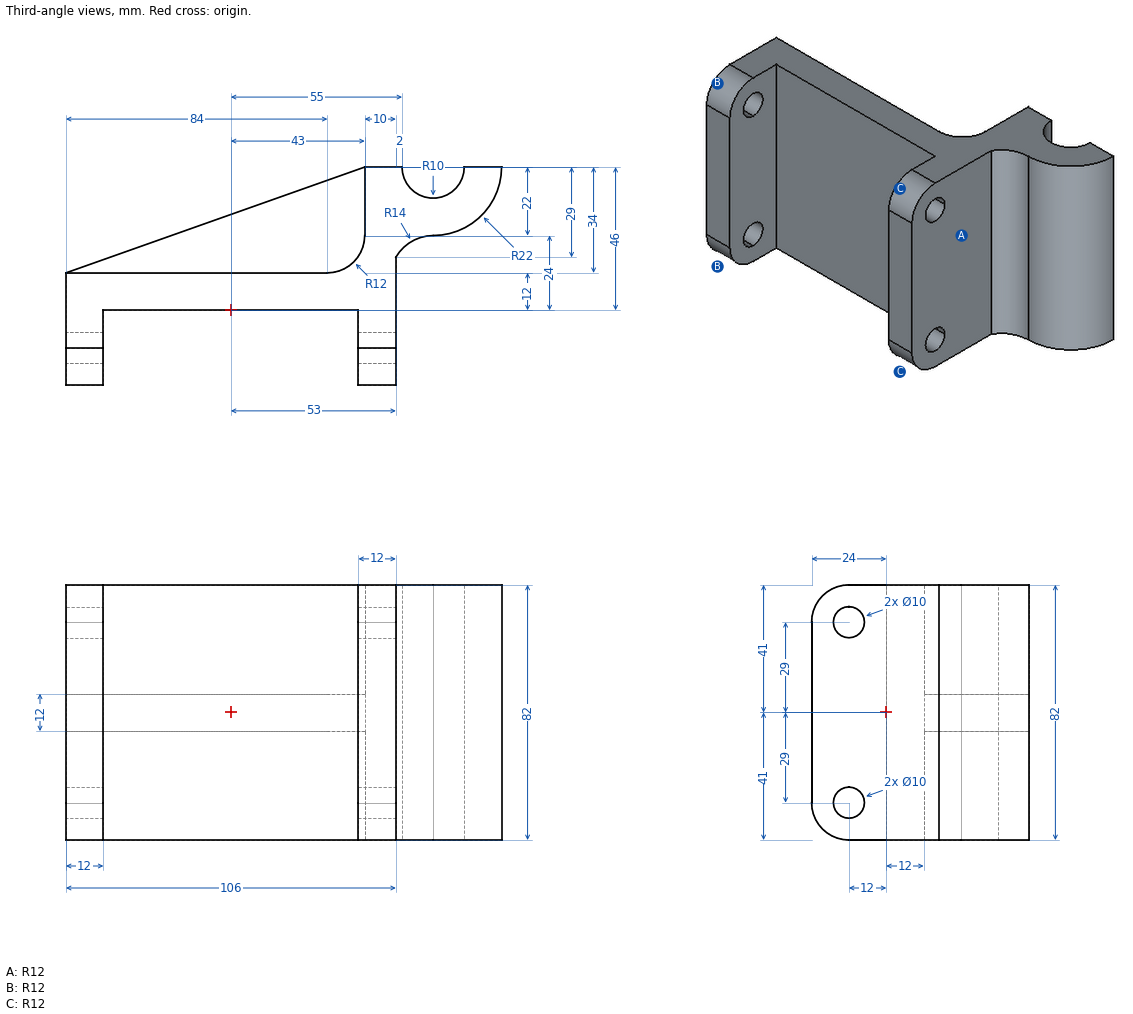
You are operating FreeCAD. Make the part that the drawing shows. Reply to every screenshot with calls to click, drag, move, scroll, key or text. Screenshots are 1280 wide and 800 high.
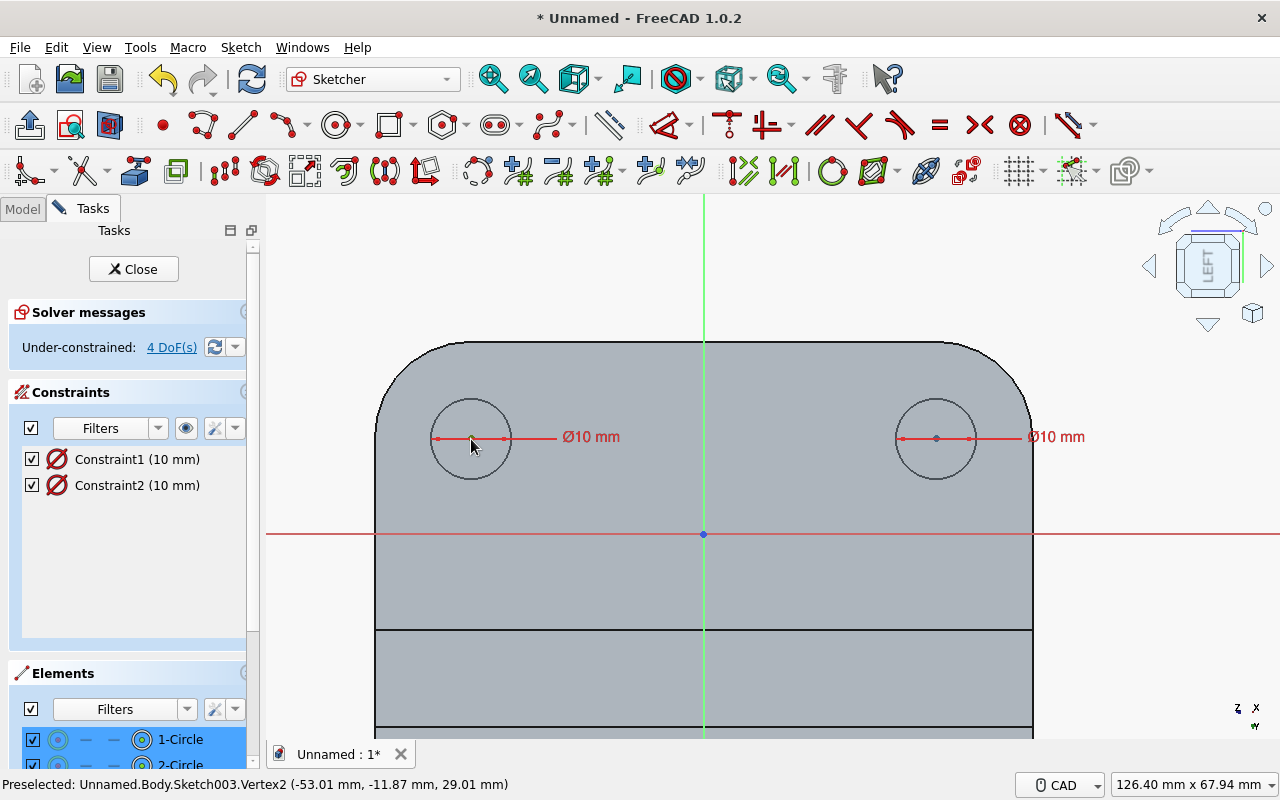
key(h)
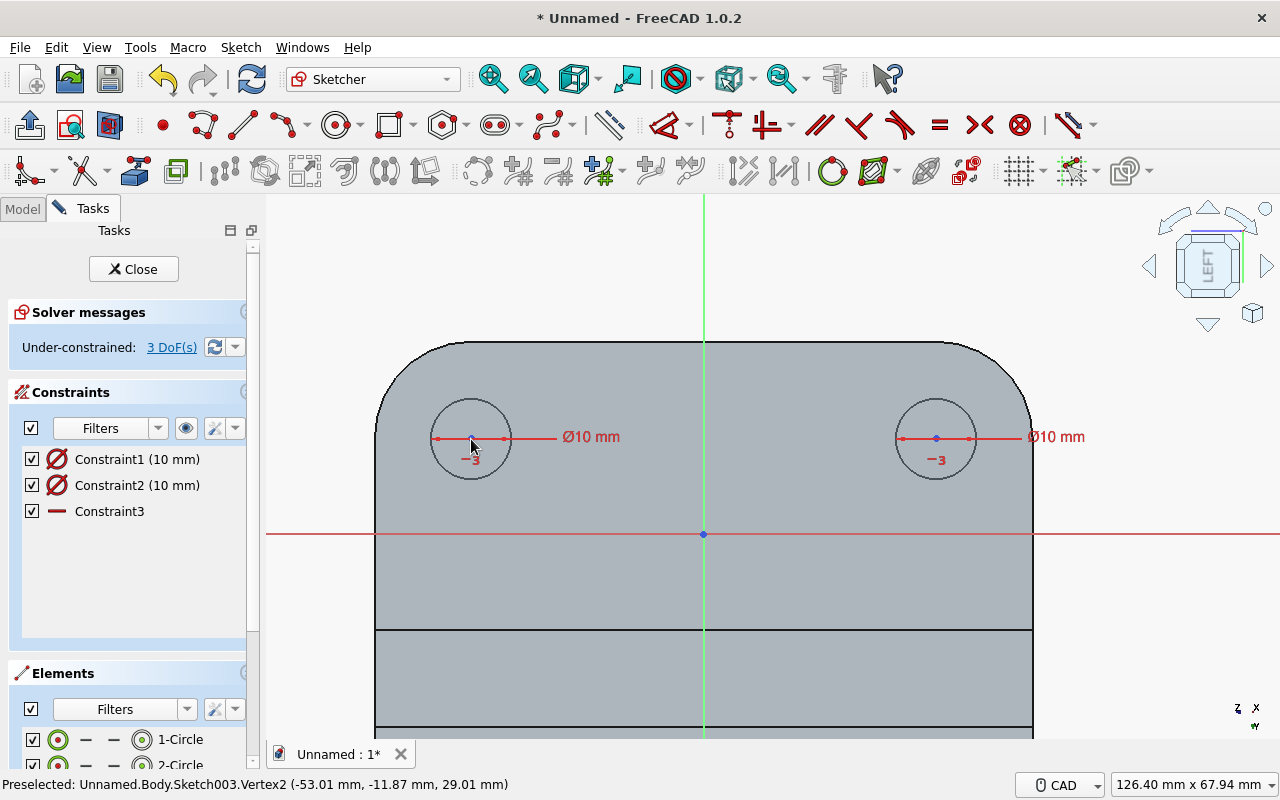
key(d)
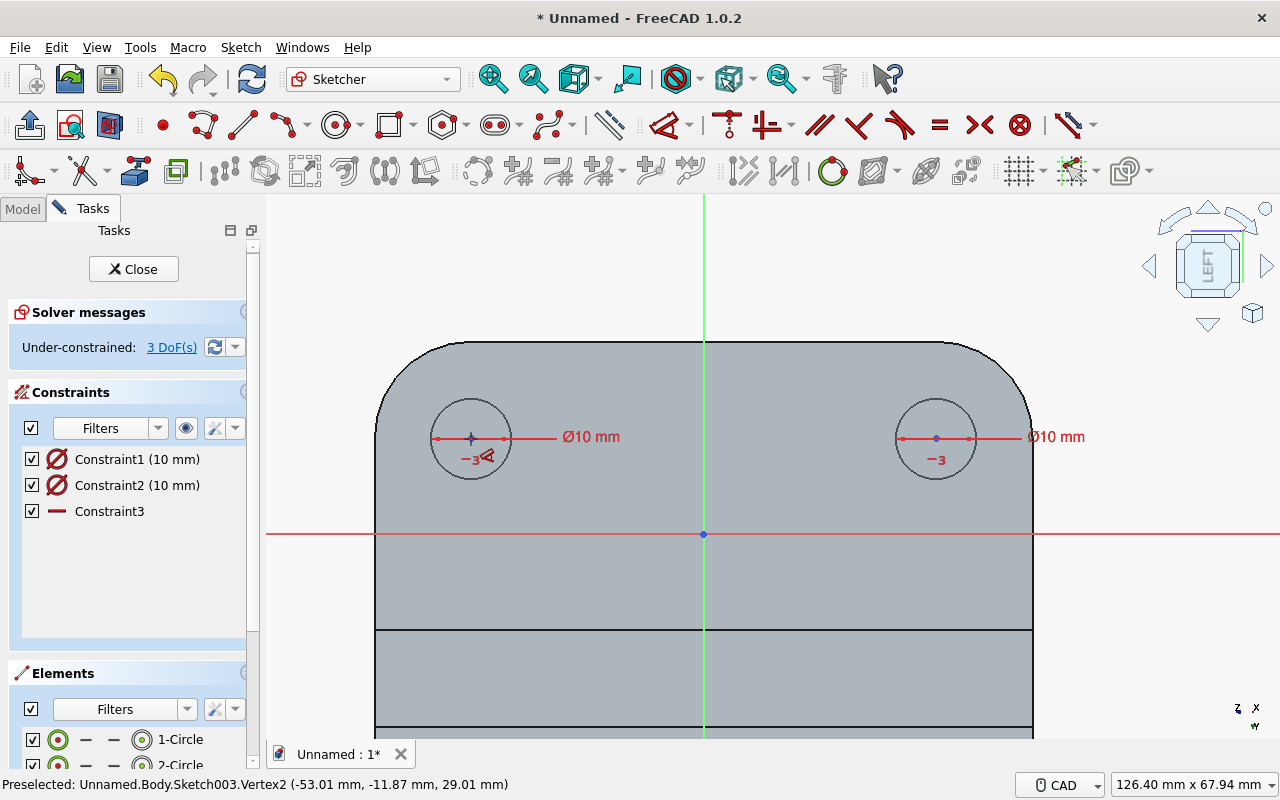
click(936, 439)
click(820, 568)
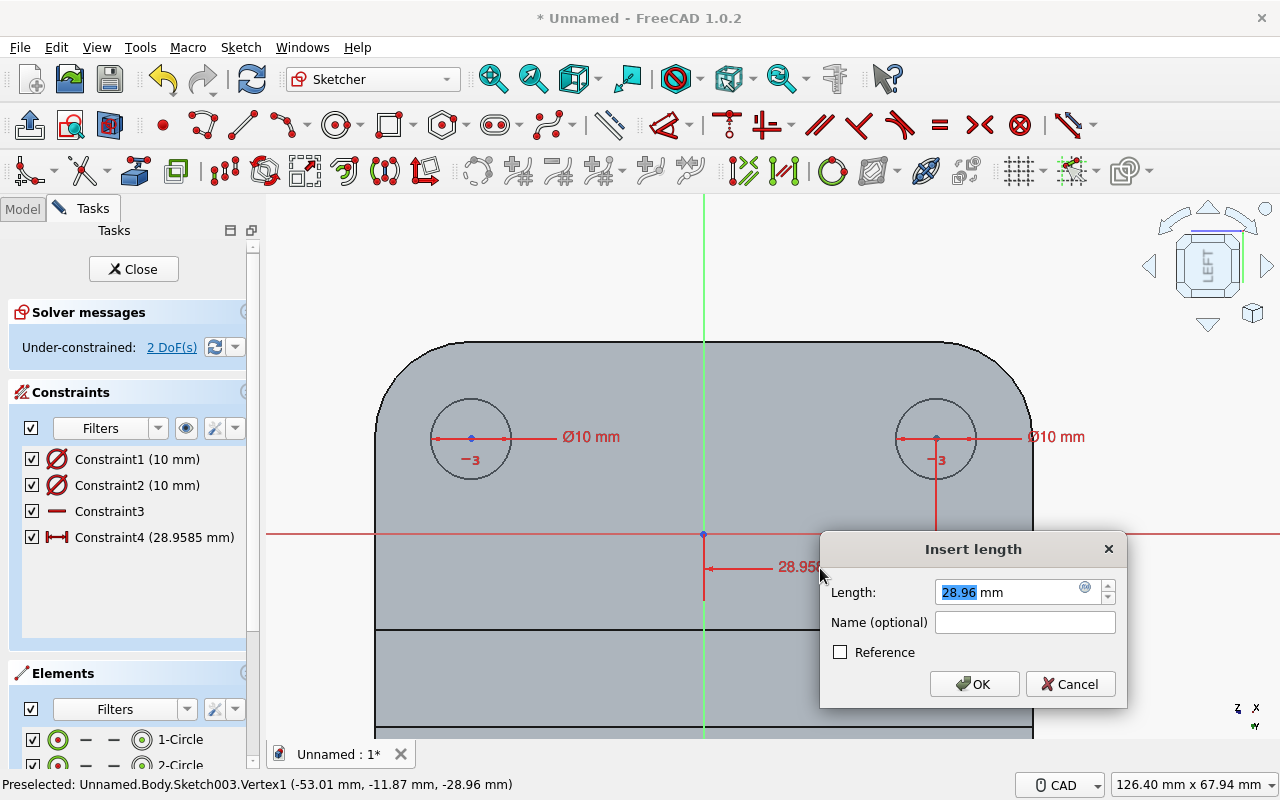
text(29)
key(Return)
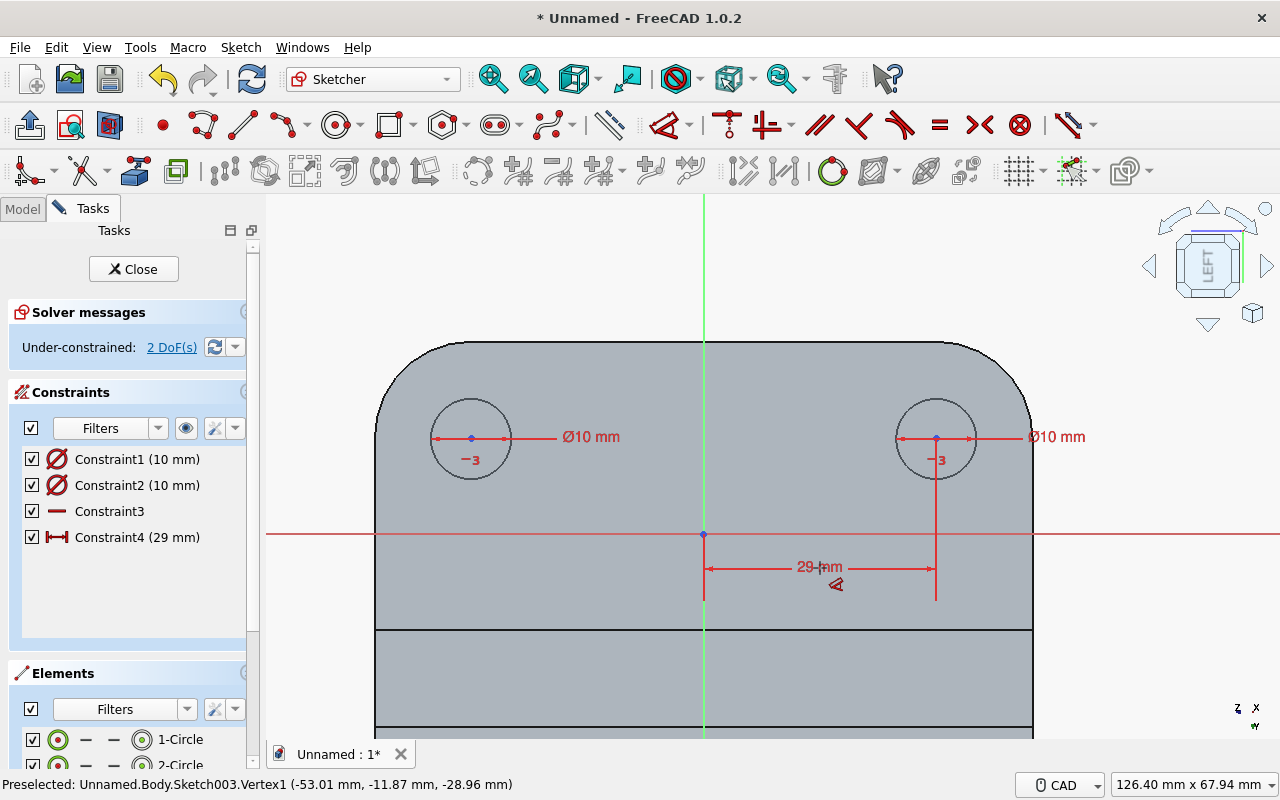
click(936, 439)
click(970, 487)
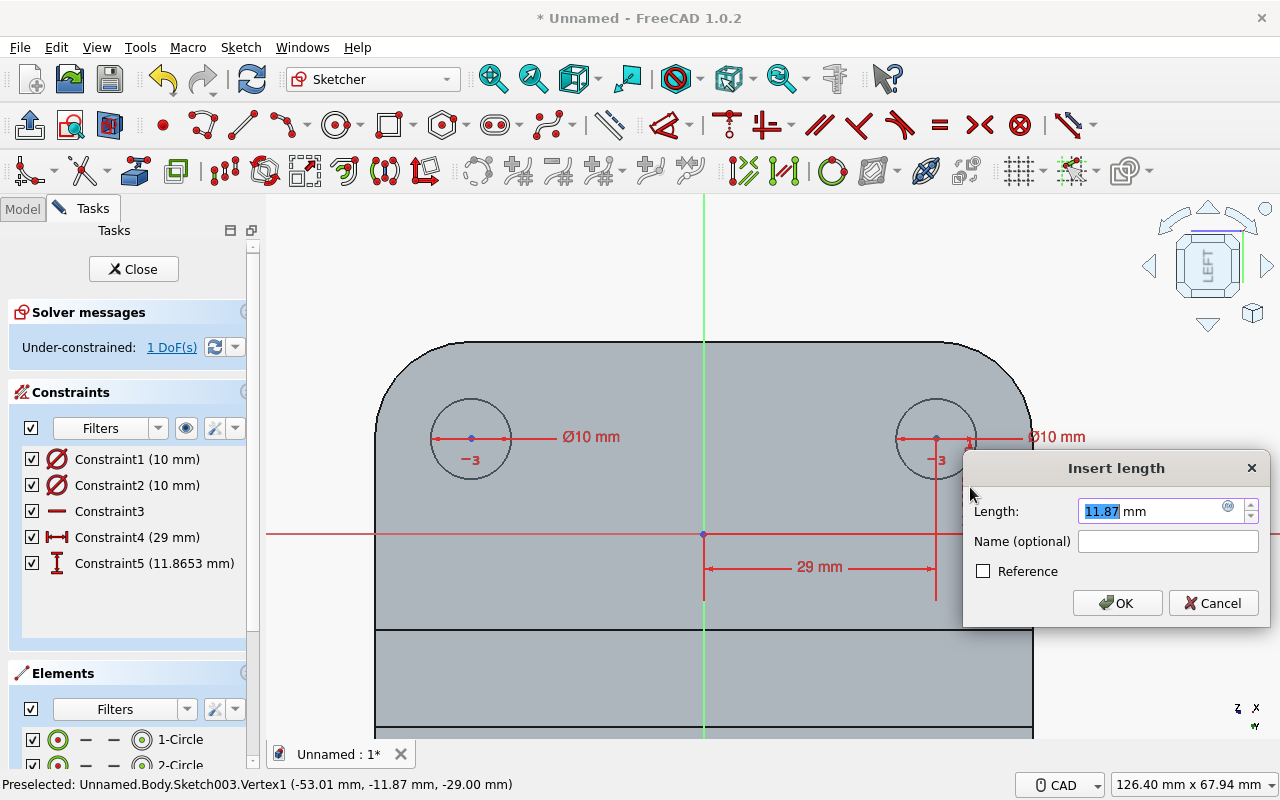
text(12)
key(Return)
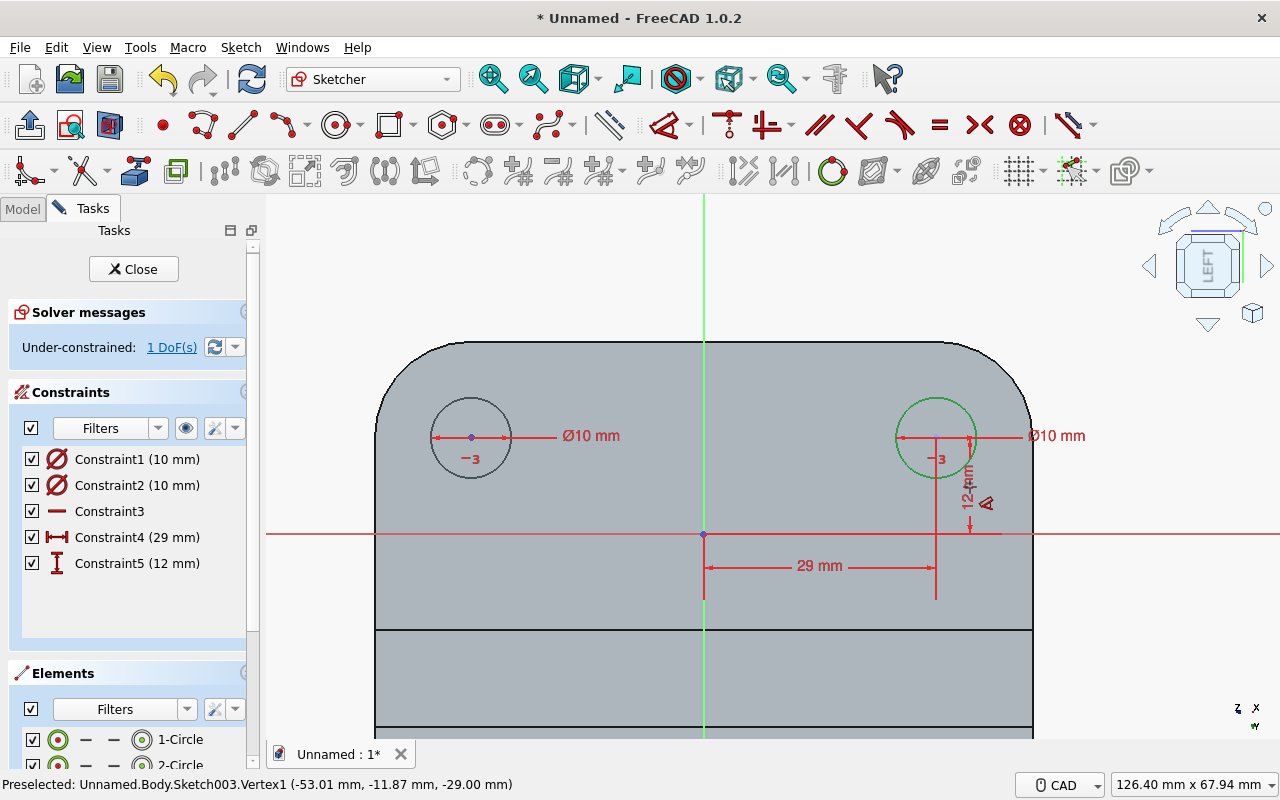
click(471, 438)
click(587, 568)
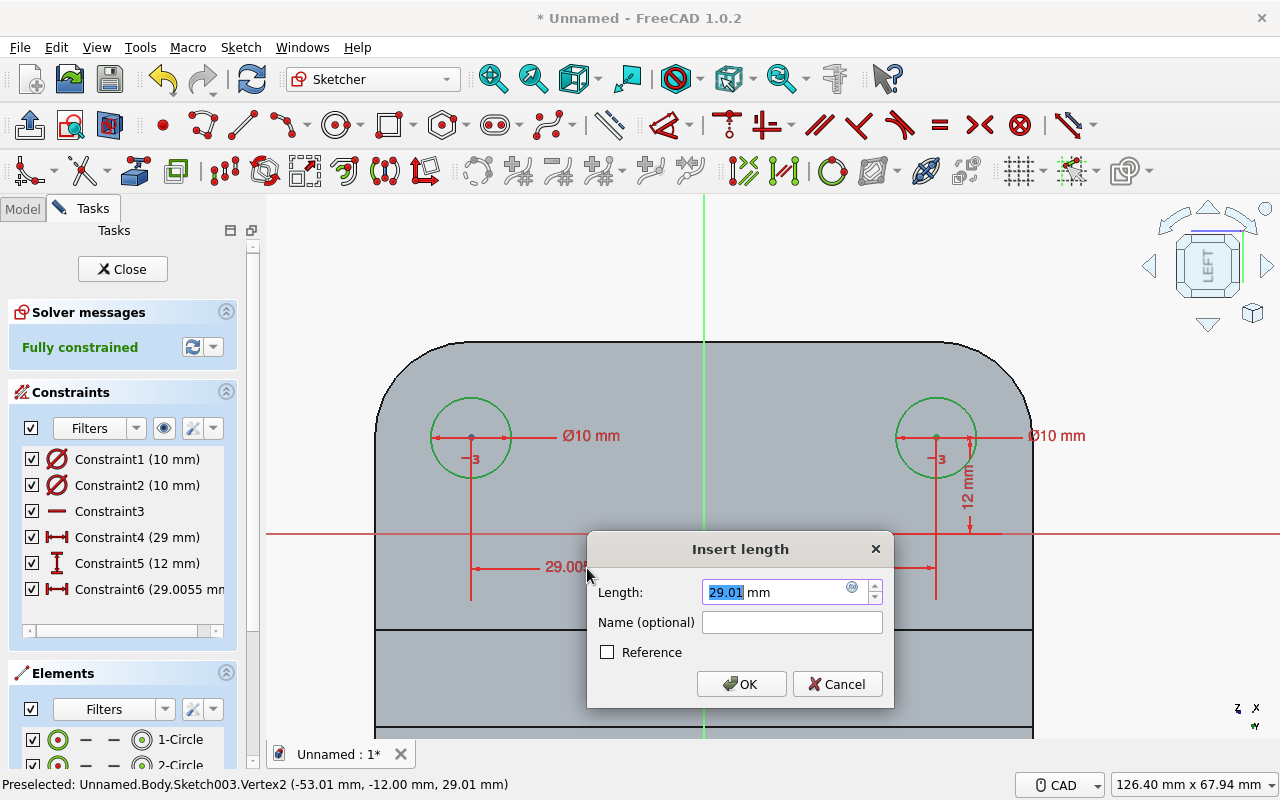
text(29)
key(Return)
key(Escape)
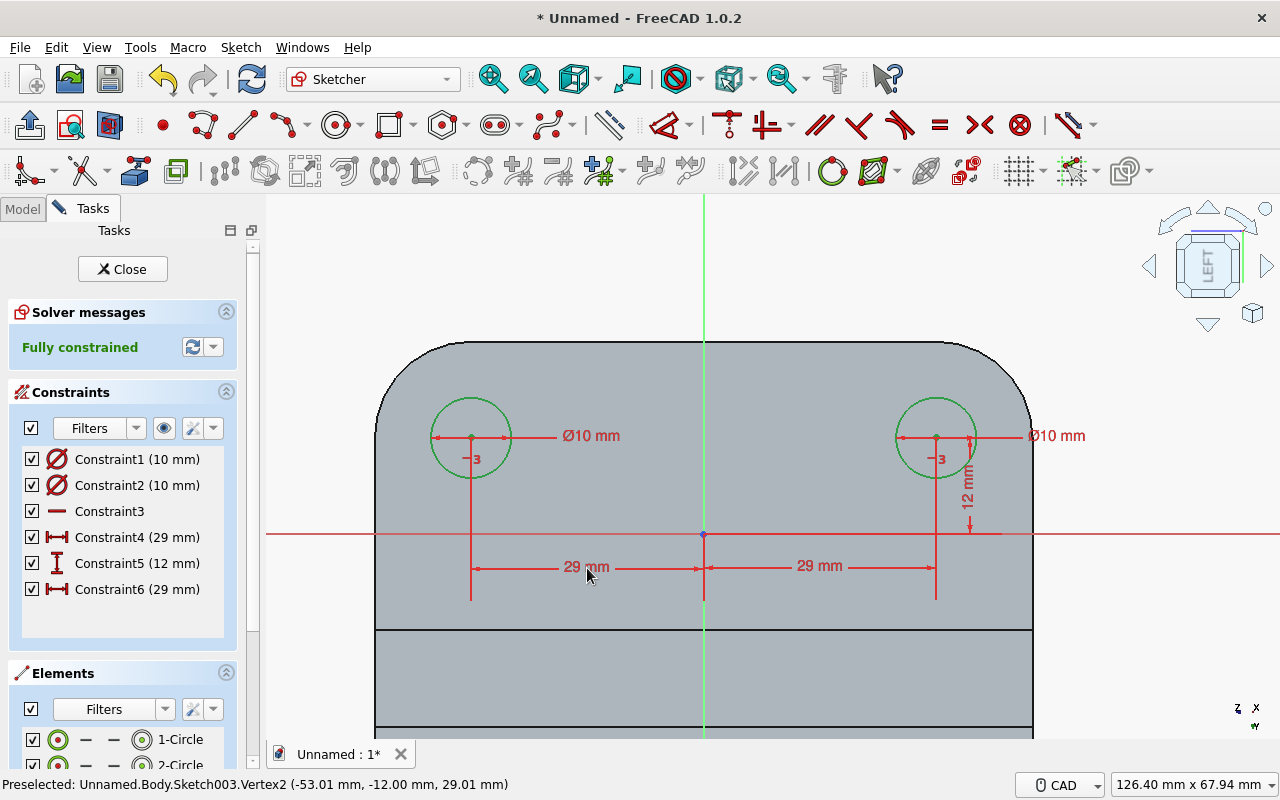
click(123, 269)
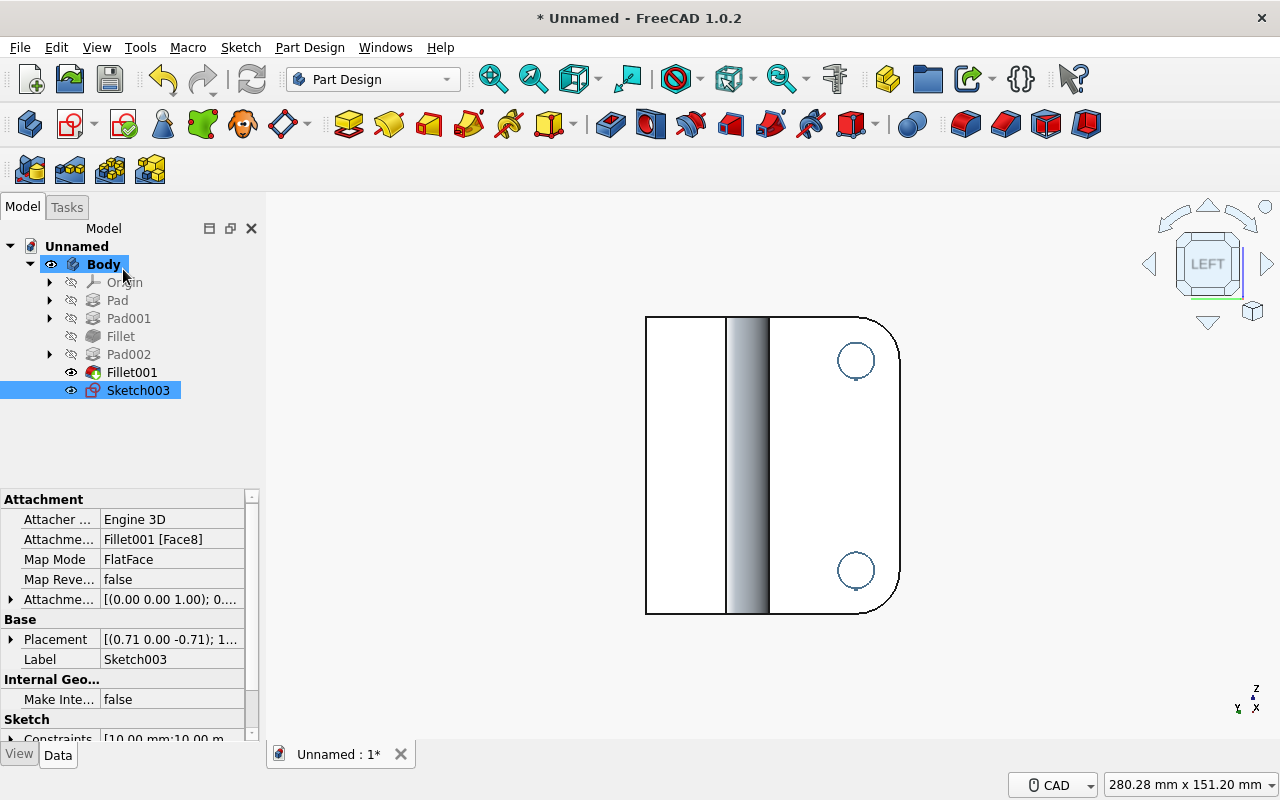
click(612, 124)